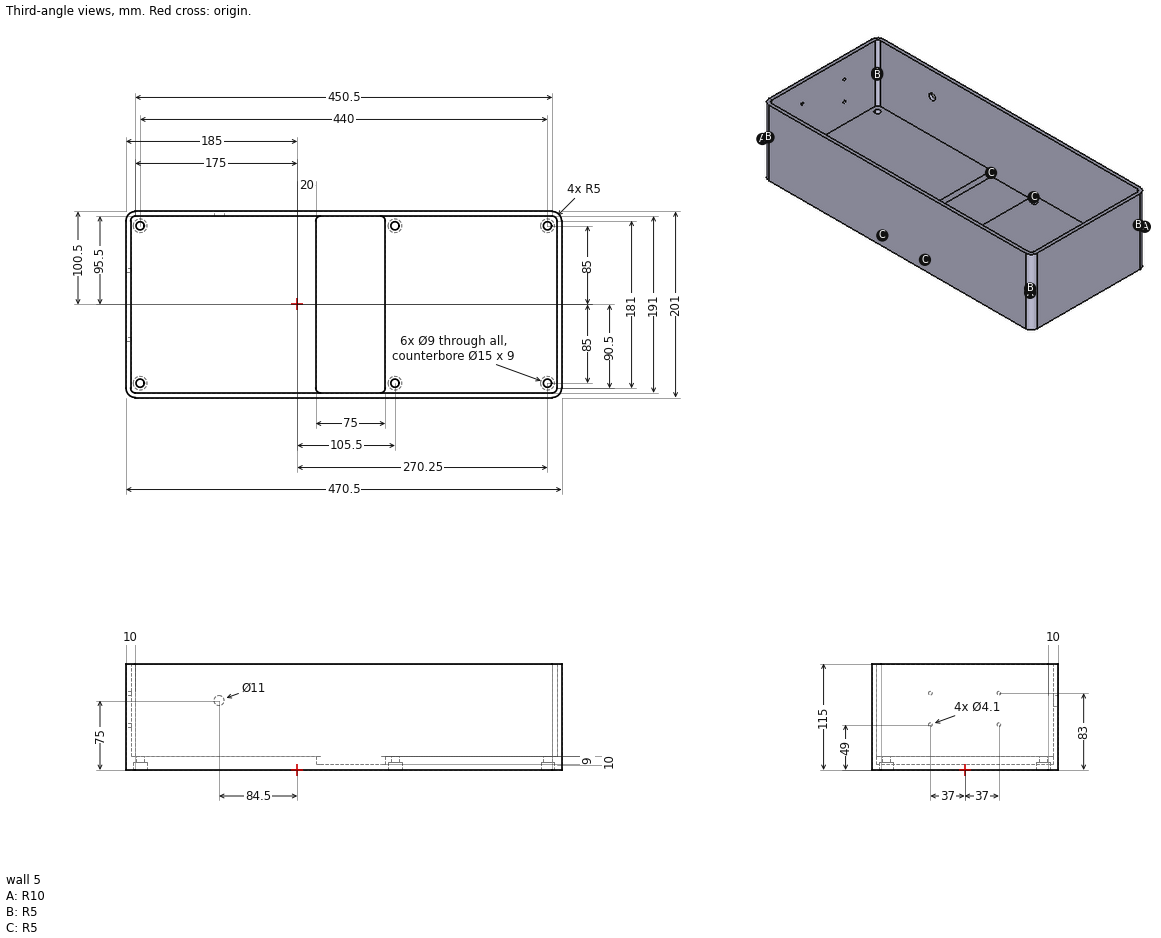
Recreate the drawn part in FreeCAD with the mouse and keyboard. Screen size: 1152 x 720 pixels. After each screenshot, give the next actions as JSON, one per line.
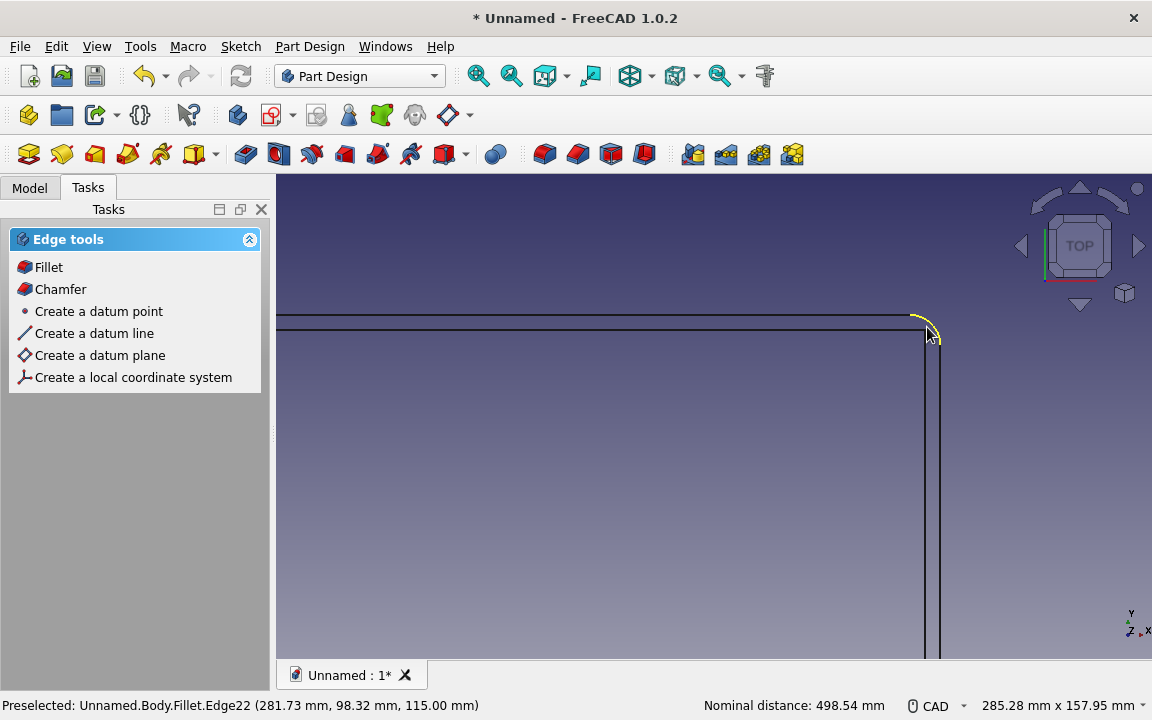
{"action": "key", "text": "v f"}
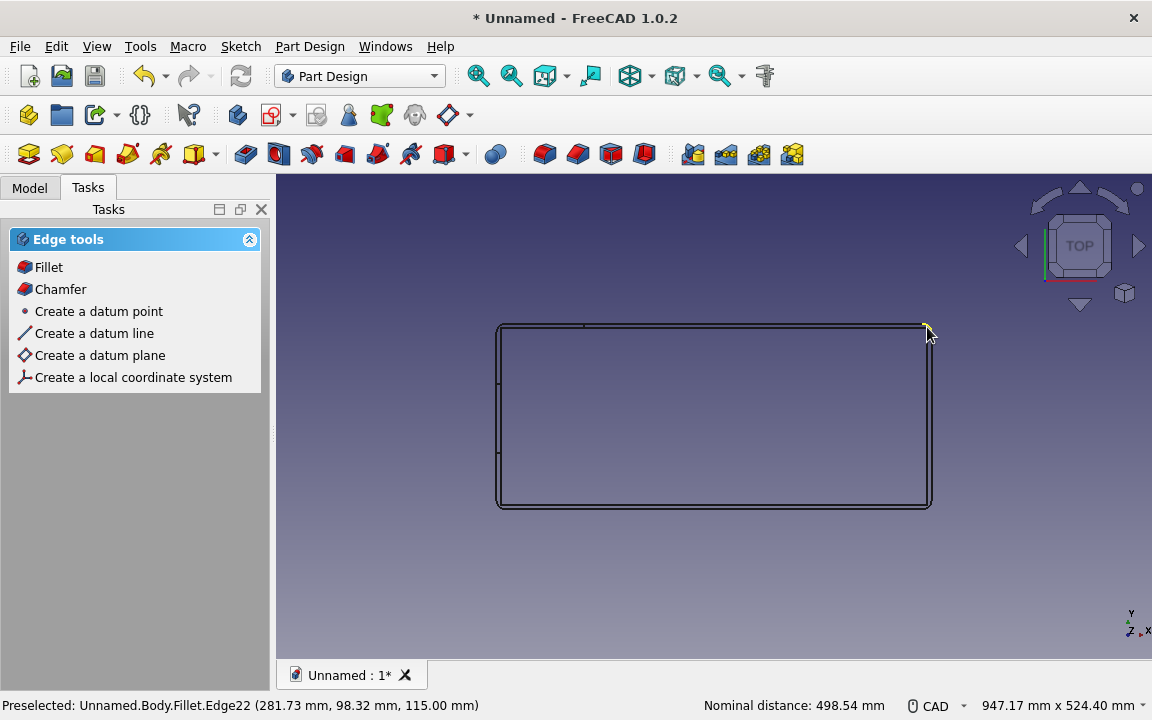
{"action": "key", "text": "1"}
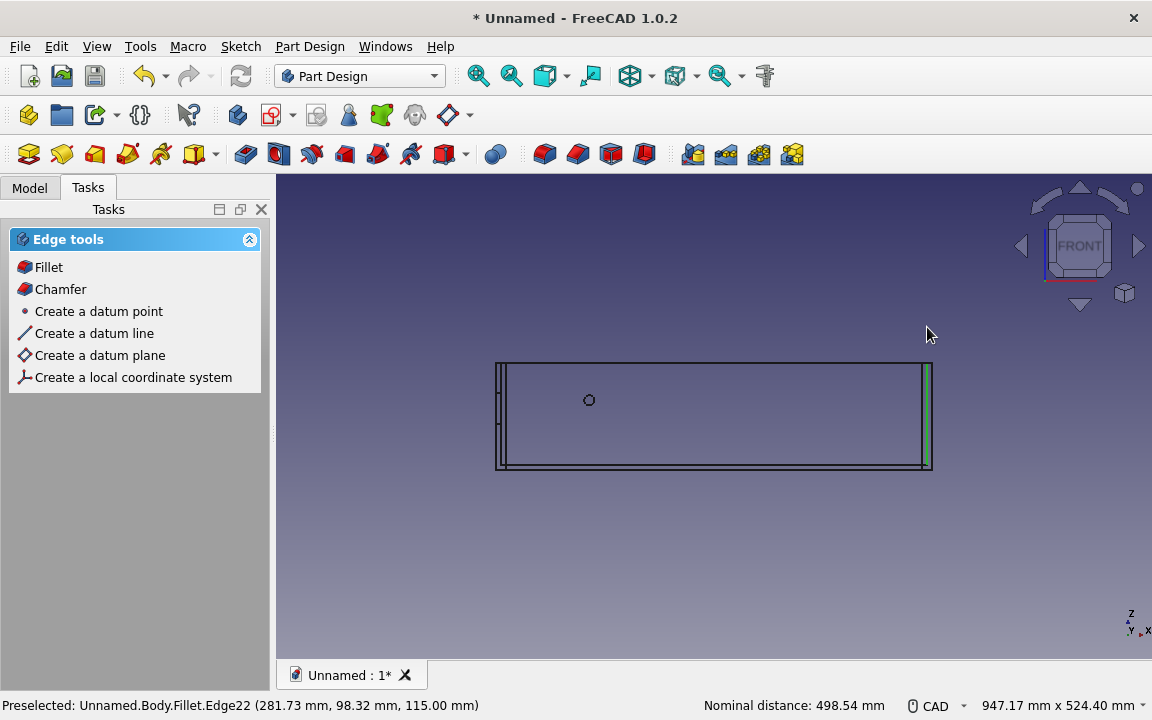
{"action": "scroll", "coordinate": [927, 413], "scroll_direction": "up", "scroll_amount": 6}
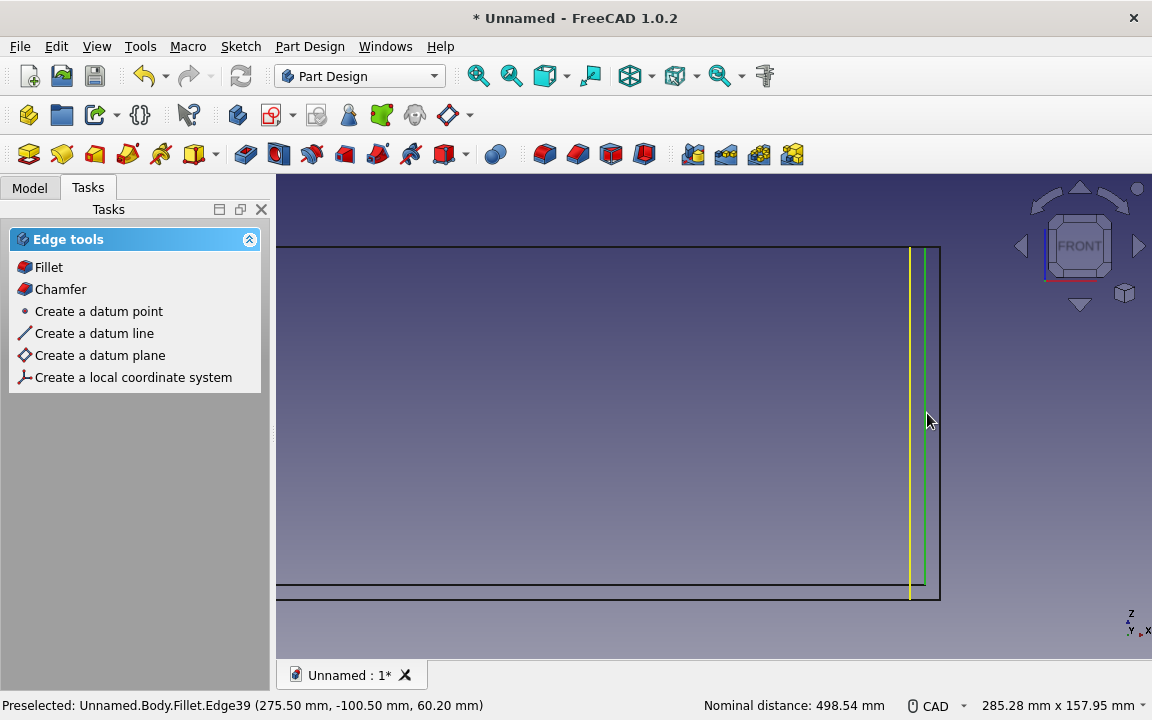
{"action": "key", "text": "v f"}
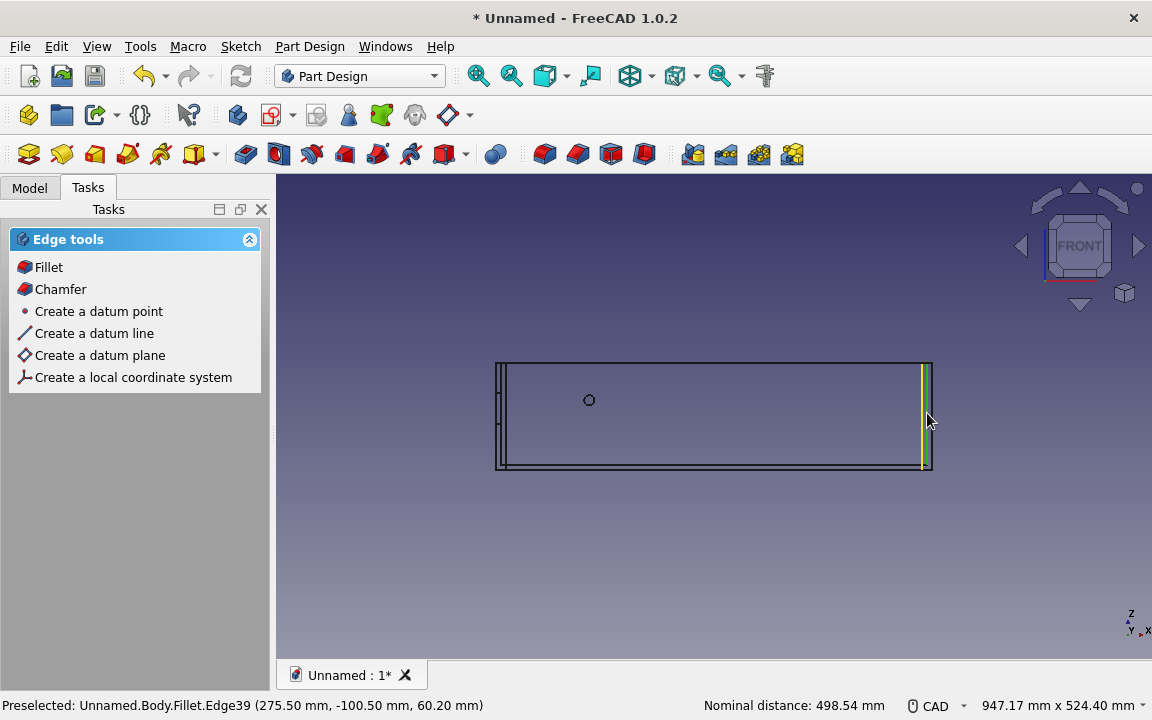
{"action": "key", "text": "3"}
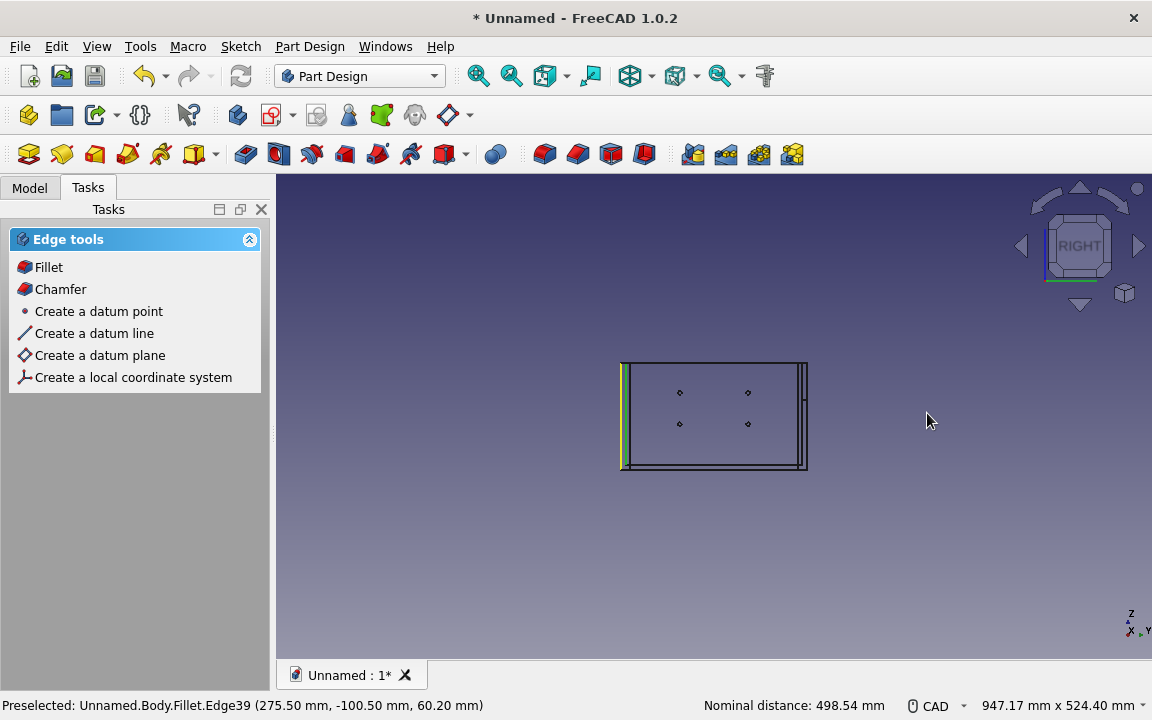
{"action": "key", "text": "v f"}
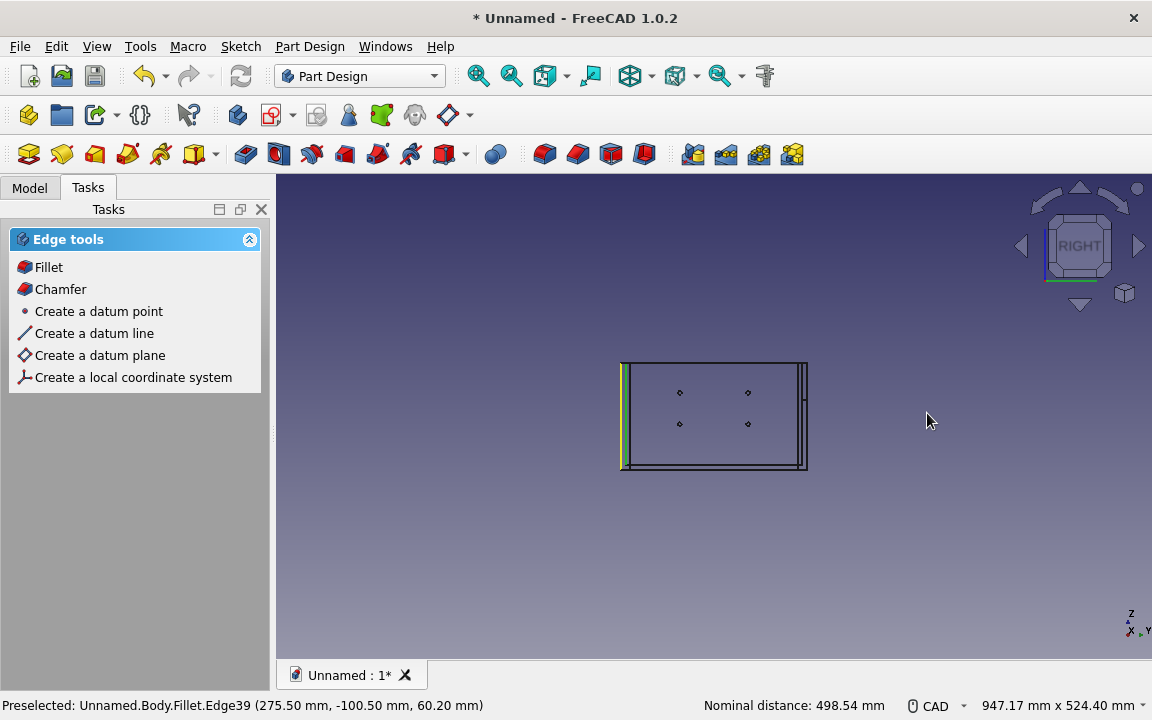
{"action": "scroll", "coordinate": [802, 413], "scroll_direction": "up", "scroll_amount": 6}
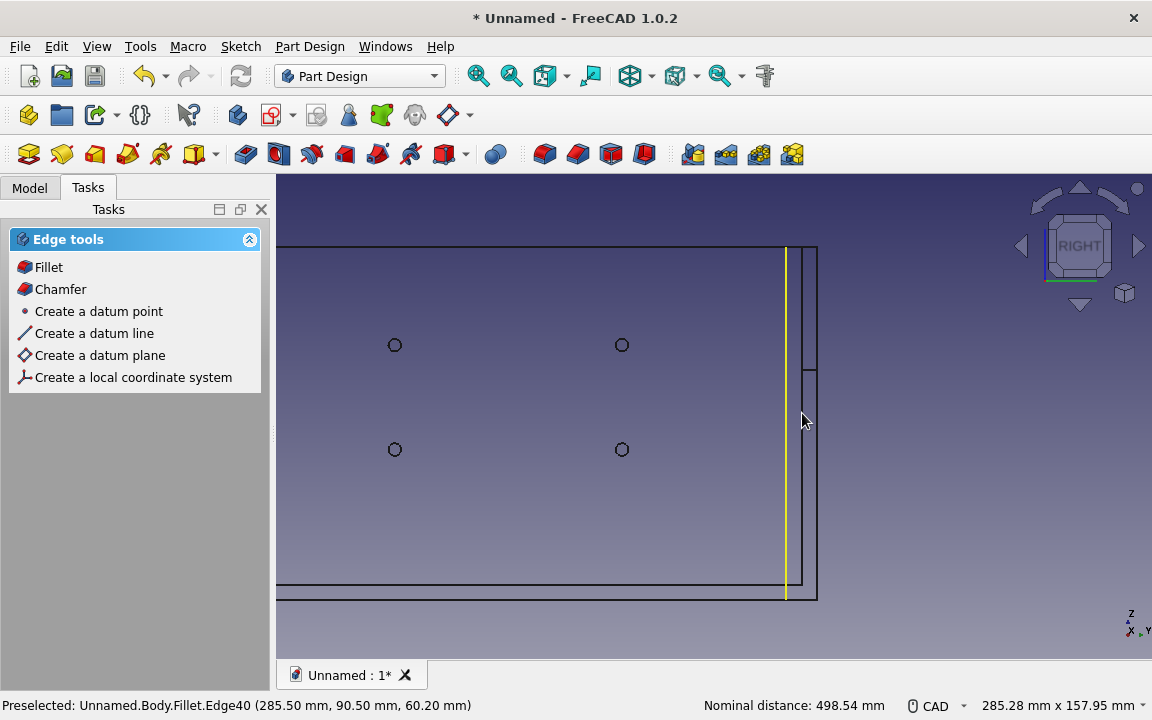
{"action": "left_click", "coordinate": [802, 415], "text": "ctrl"}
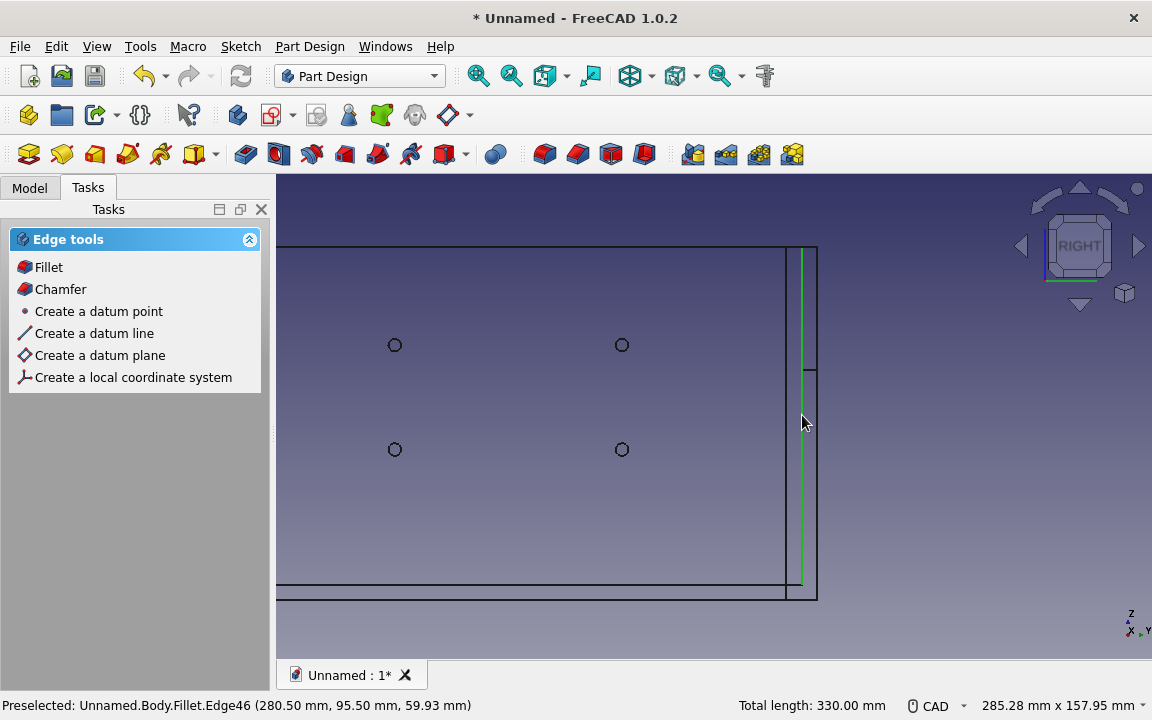
{"action": "left_click", "coordinate": [479, 76]}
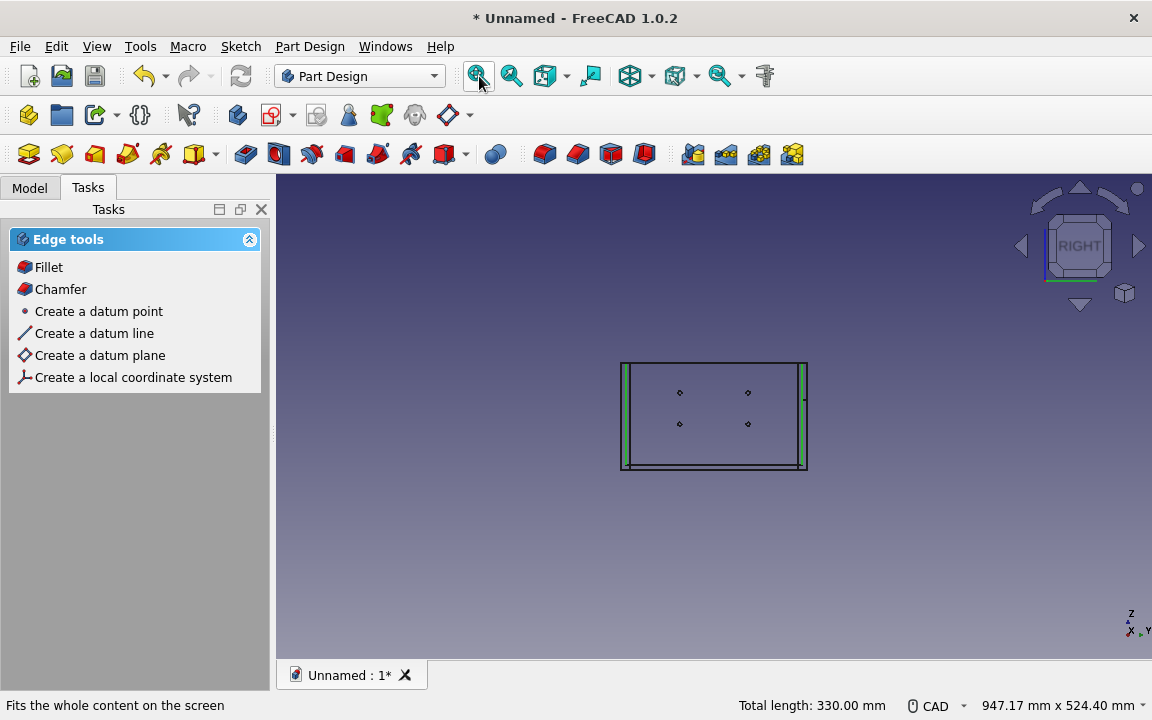
{"action": "key", "text": "5"}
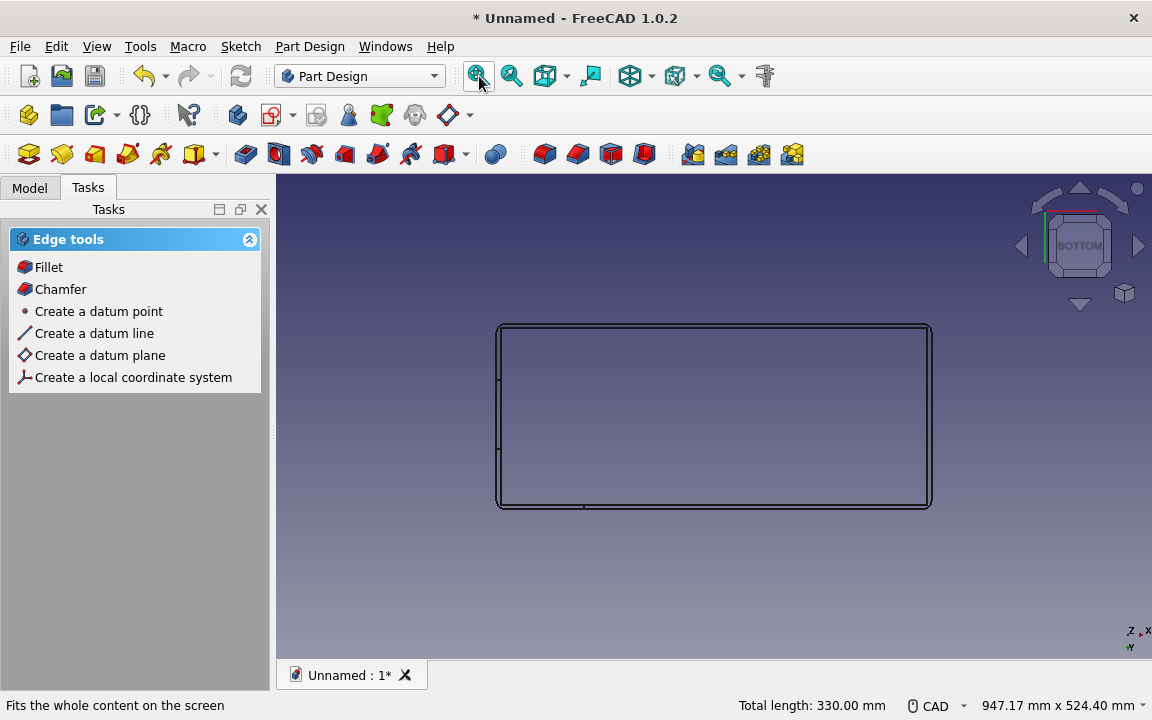
{"action": "scroll", "coordinate": [501, 327], "scroll_direction": "up", "scroll_amount": 6}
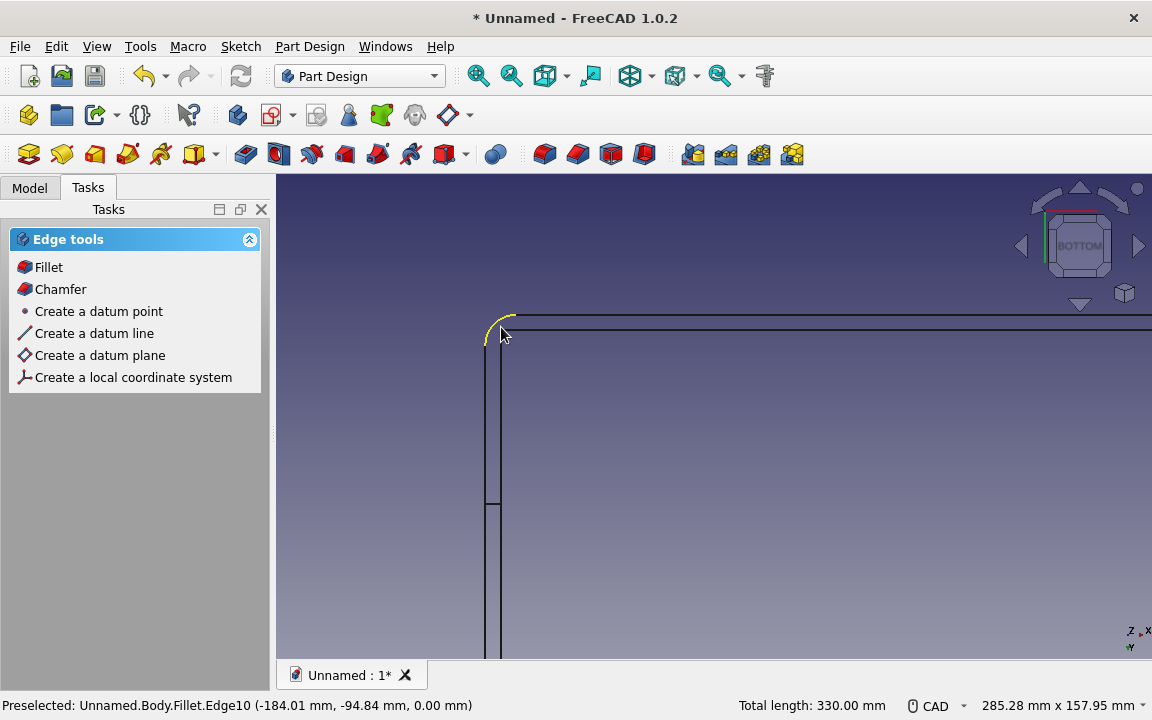
{"action": "key", "text": "v f"}